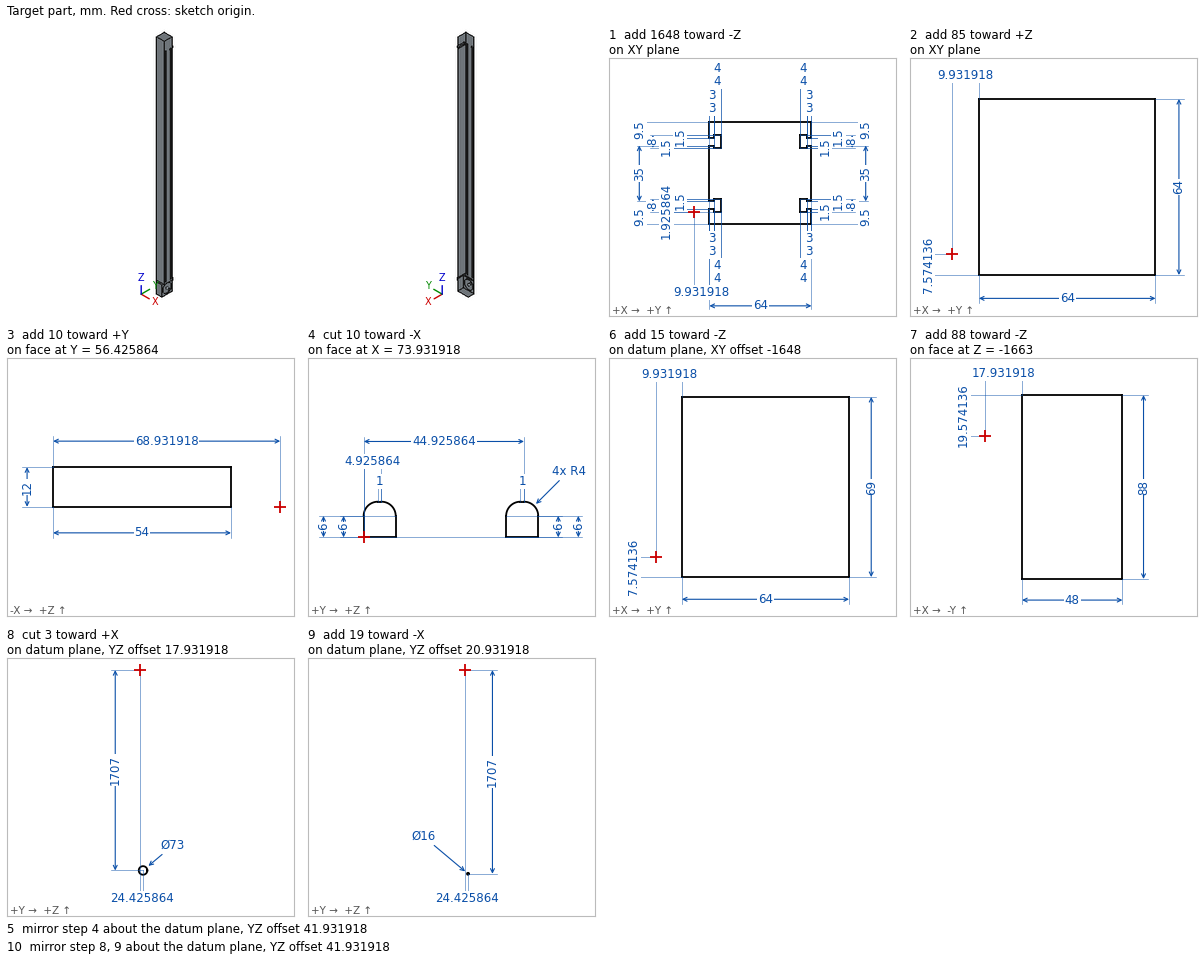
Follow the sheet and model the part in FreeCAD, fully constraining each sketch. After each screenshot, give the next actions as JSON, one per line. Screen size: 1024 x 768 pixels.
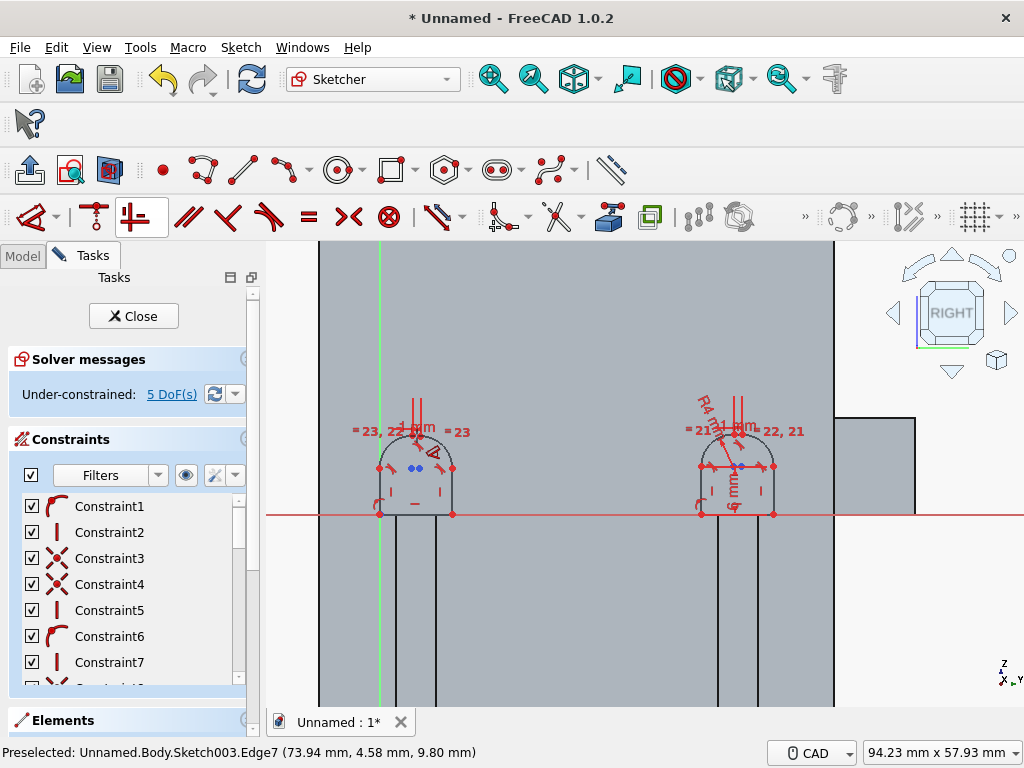
{"action": "left_click", "coordinate": [380, 482]}
{"action": "left_click", "coordinate": [346, 491]}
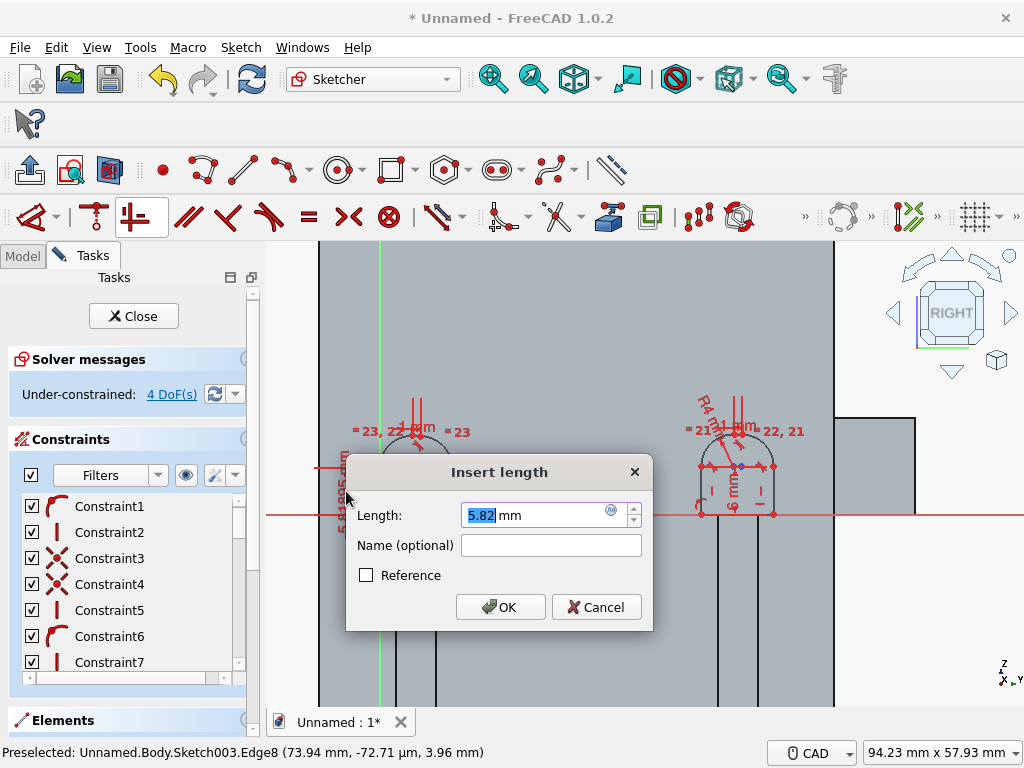
{"action": "type", "text": "6"}
{"action": "key", "text": "Return"}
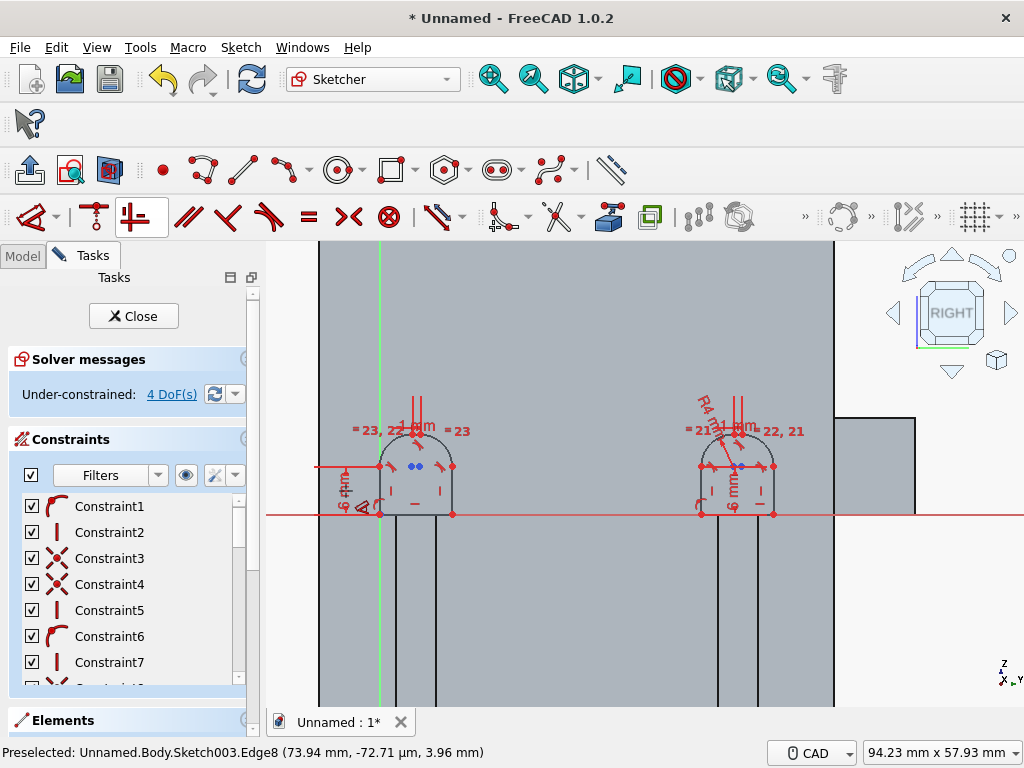
{"action": "left_click", "coordinate": [774, 467]}
{"action": "left_click", "coordinate": [808, 491]}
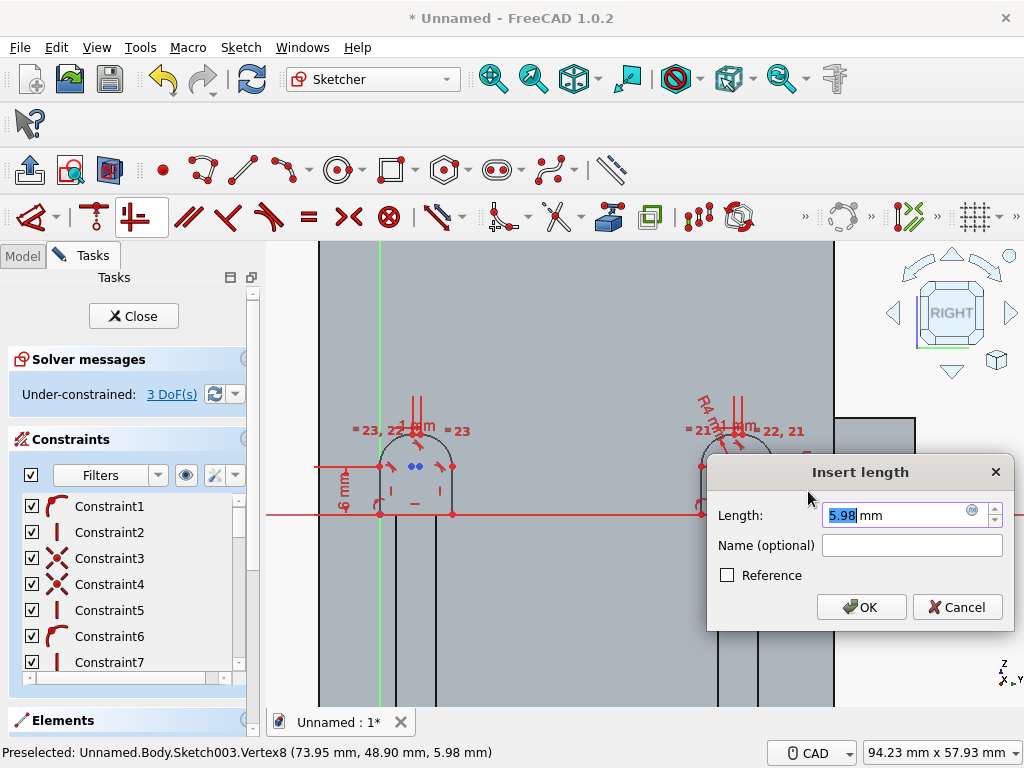
{"action": "type", "text": "6"}
{"action": "key", "text": "Return"}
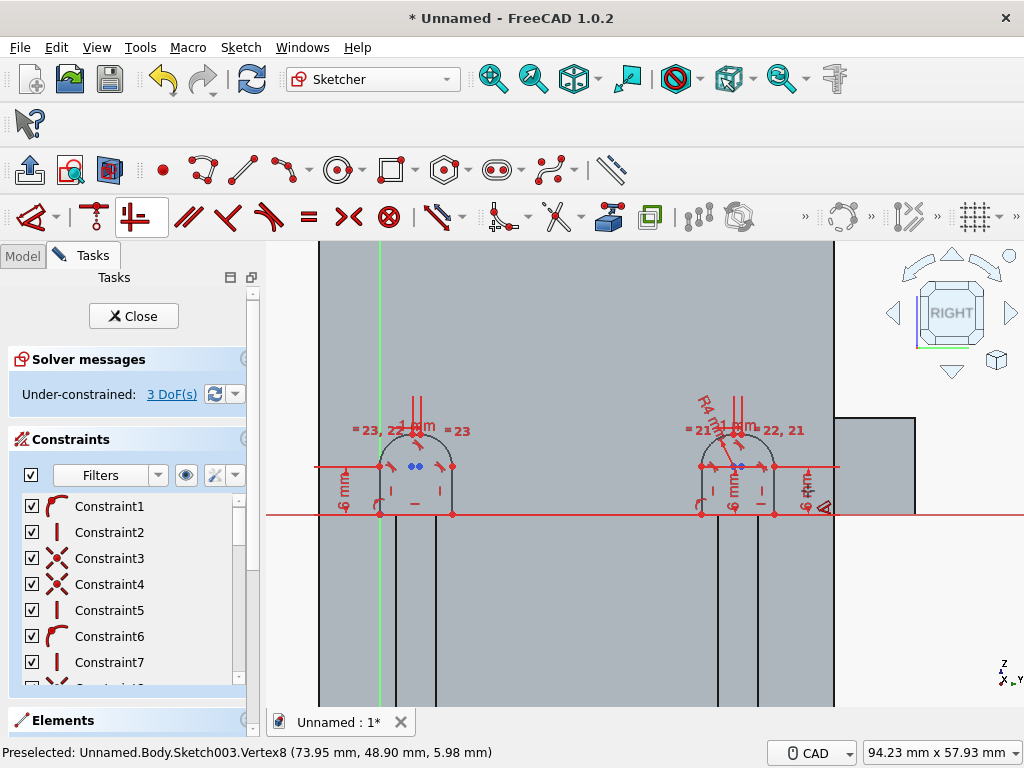
{"action": "left_click", "coordinate": [452, 467]}
{"action": "left_click", "coordinate": [486, 491]}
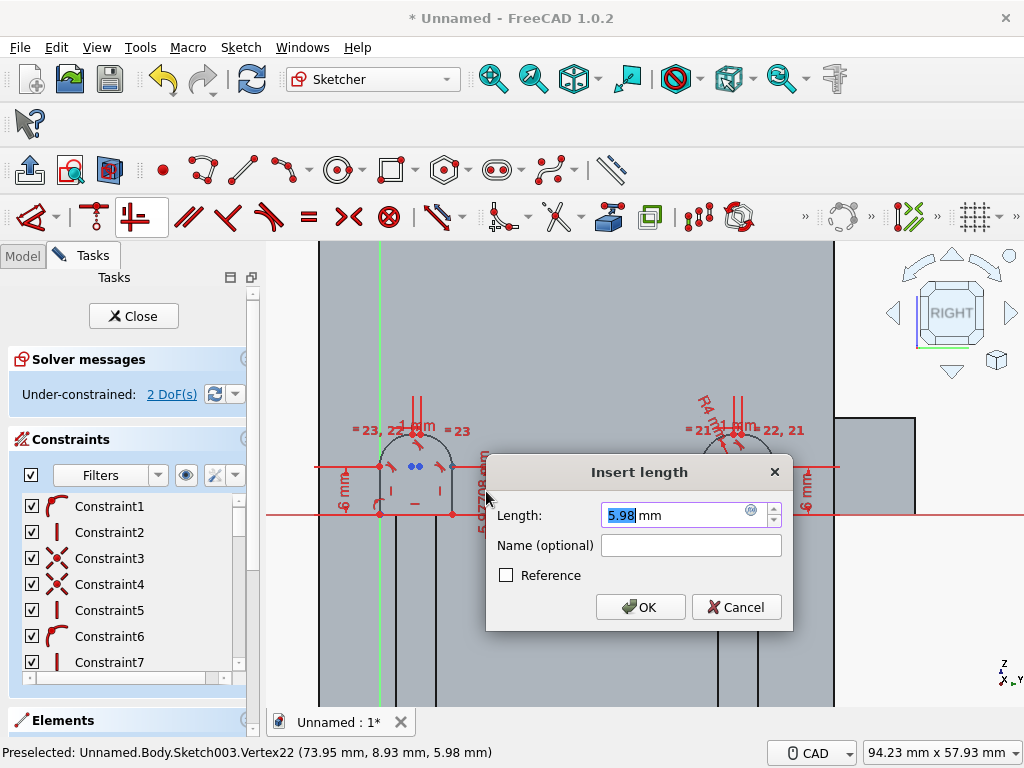
{"action": "type", "text": "6"}
{"action": "key", "text": "Return"}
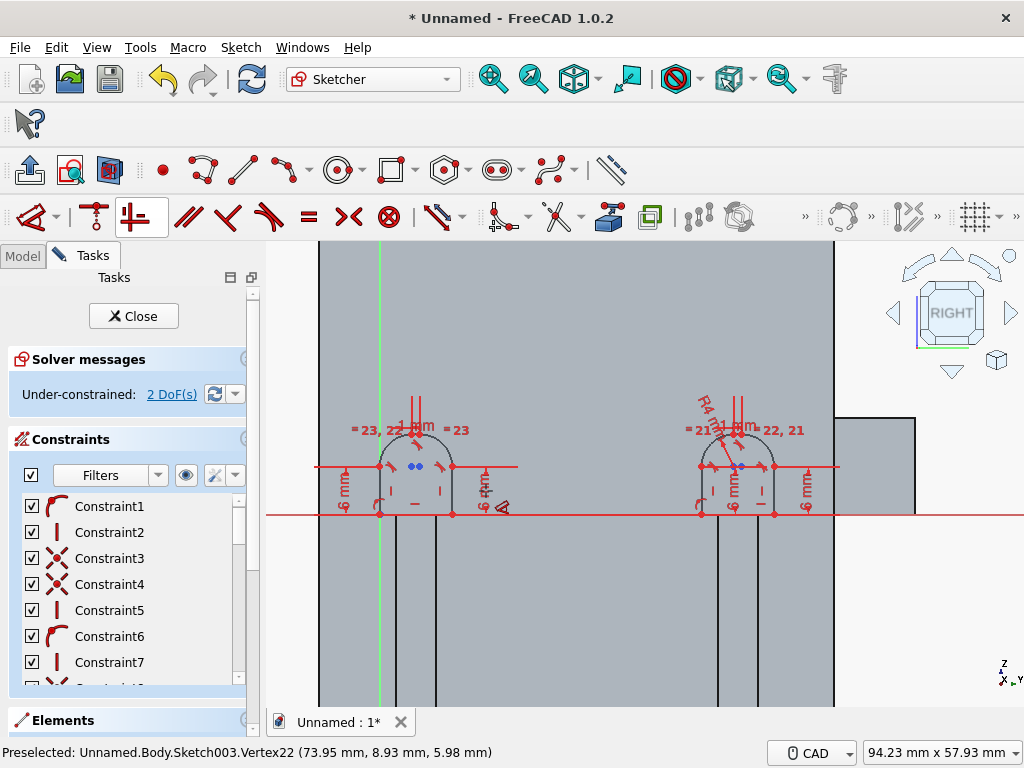
{"action": "scroll", "coordinate": [420, 434], "scroll_direction": "up", "scroll_amount": 3}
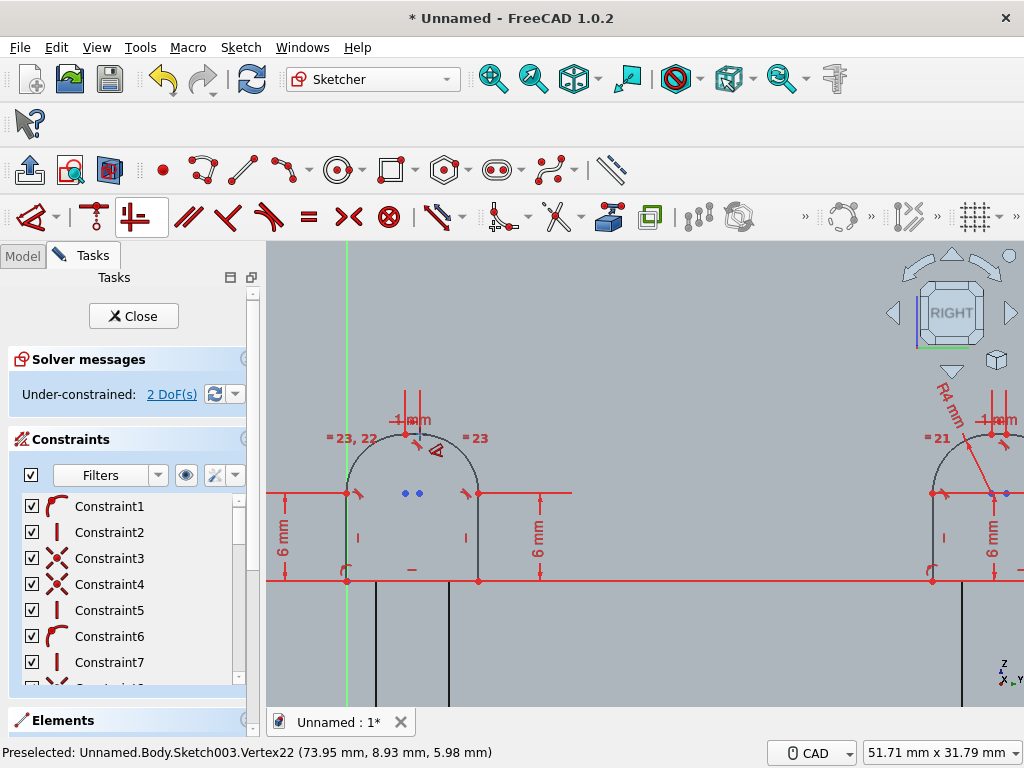
{"action": "left_click", "coordinate": [420, 434]}
{"action": "left_click", "coordinate": [384, 400]}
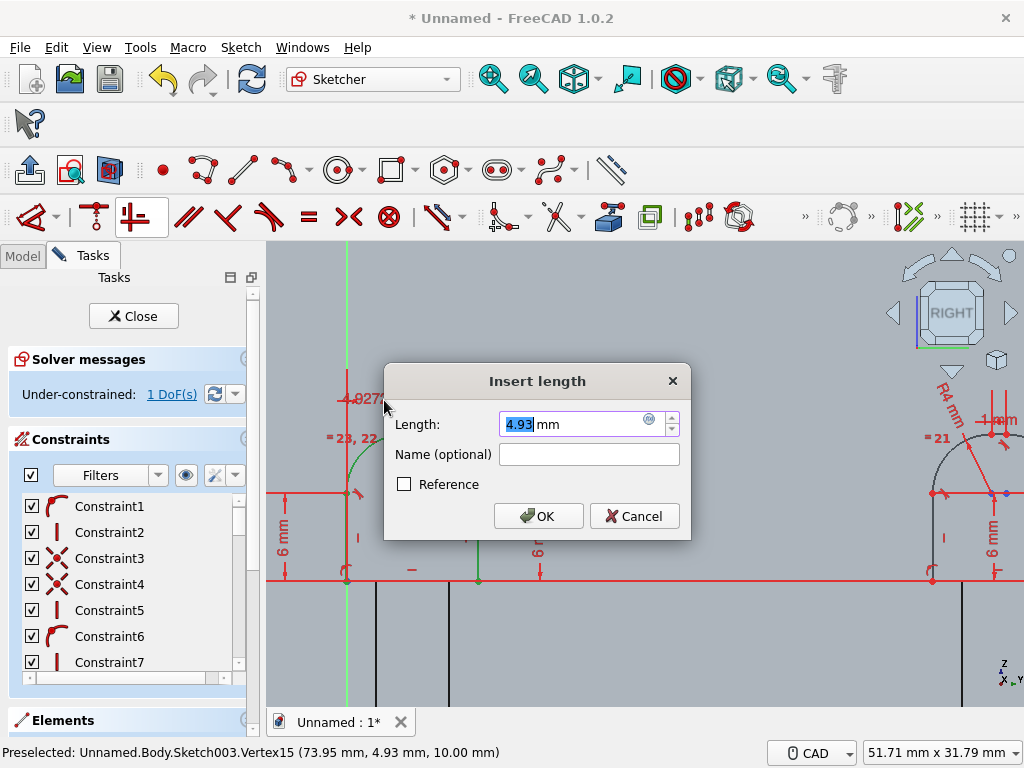
{"action": "type", "text": "4.925864"}
{"action": "key", "text": "Return"}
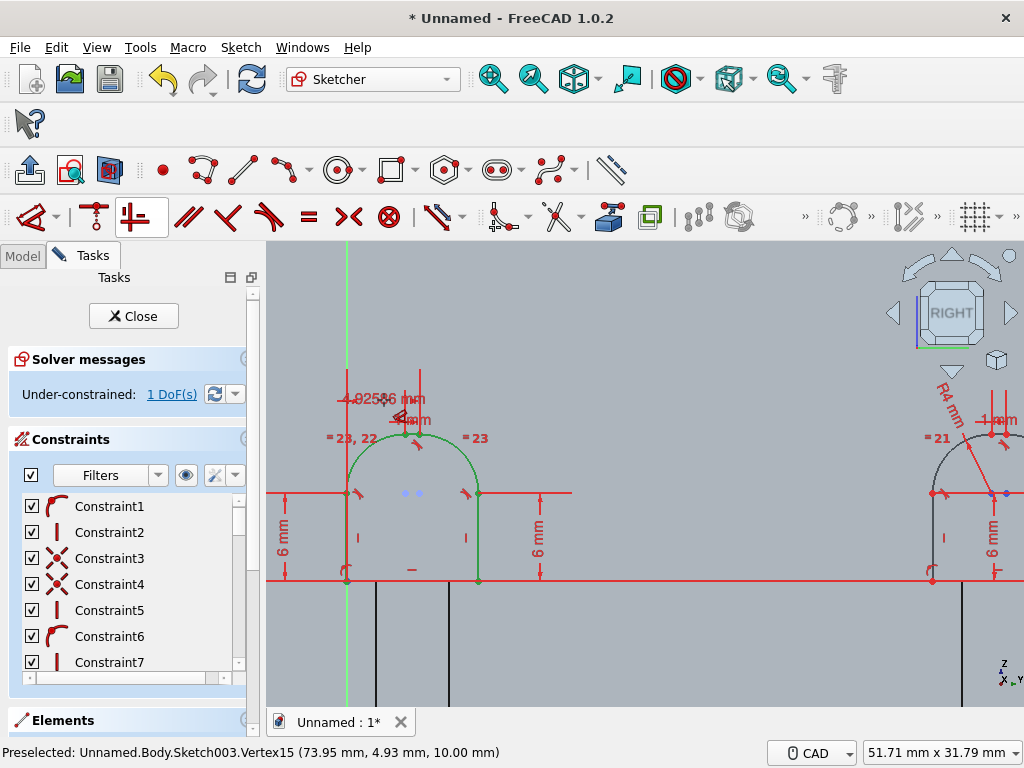
{"action": "scroll", "coordinate": [420, 433], "scroll_direction": "down", "scroll_amount": 3}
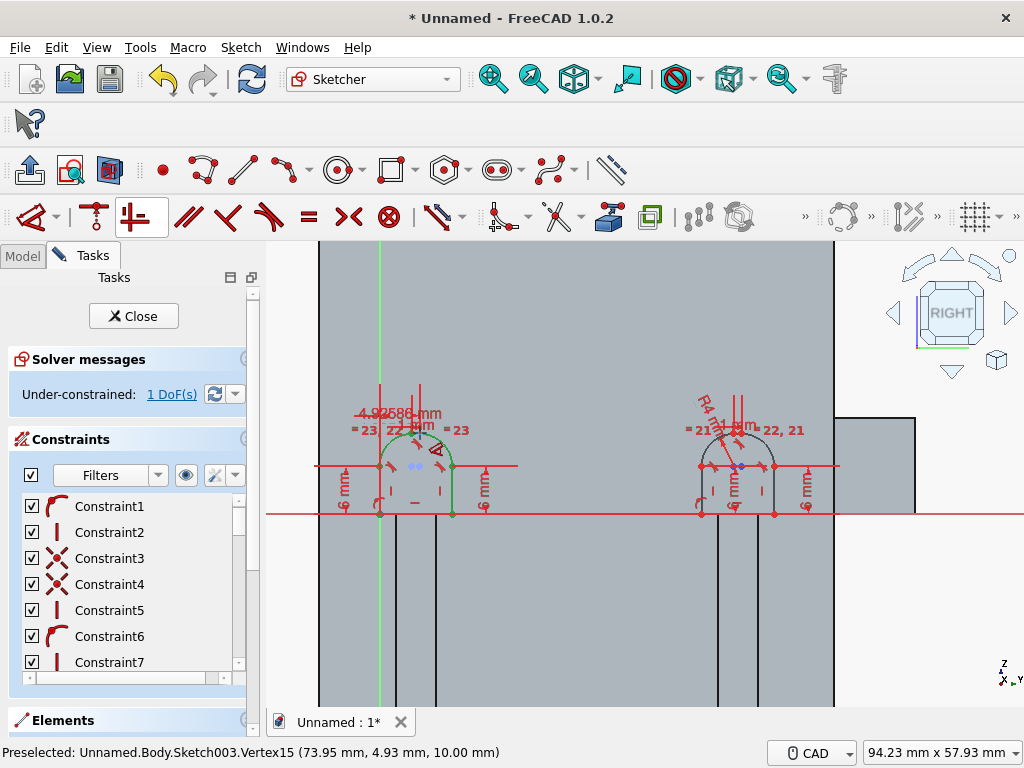
{"action": "scroll", "coordinate": [742, 434], "scroll_direction": "up", "scroll_amount": 3}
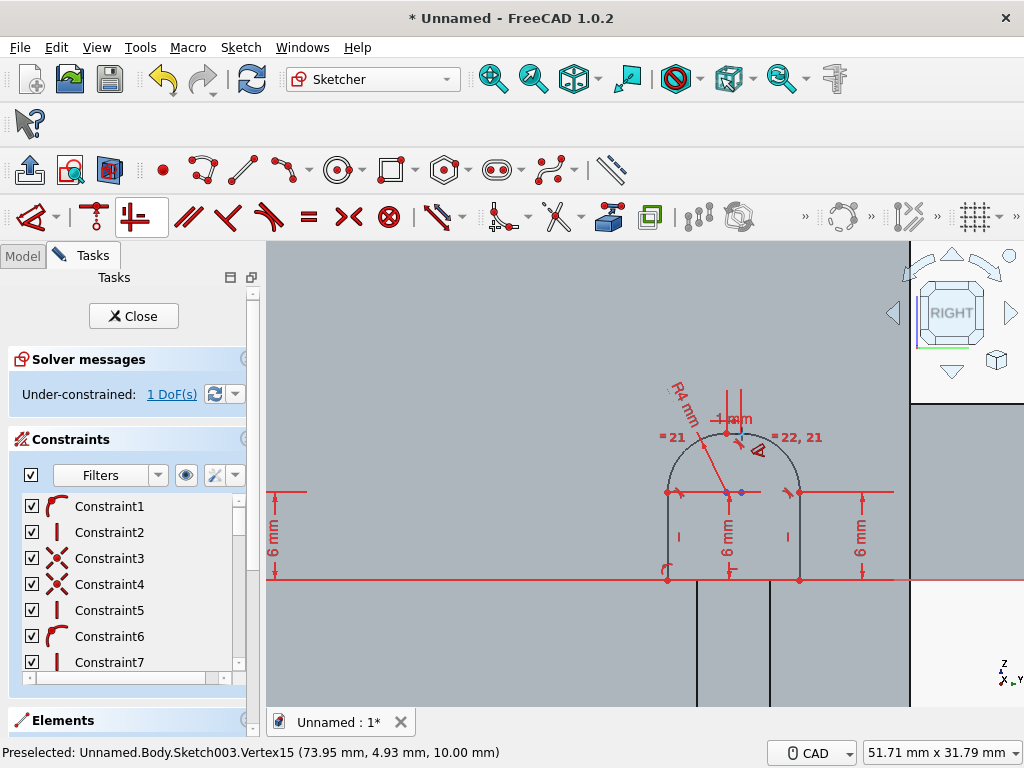
{"action": "left_click", "coordinate": [741, 434]}
{"action": "left_click", "coordinate": [518, 614]}